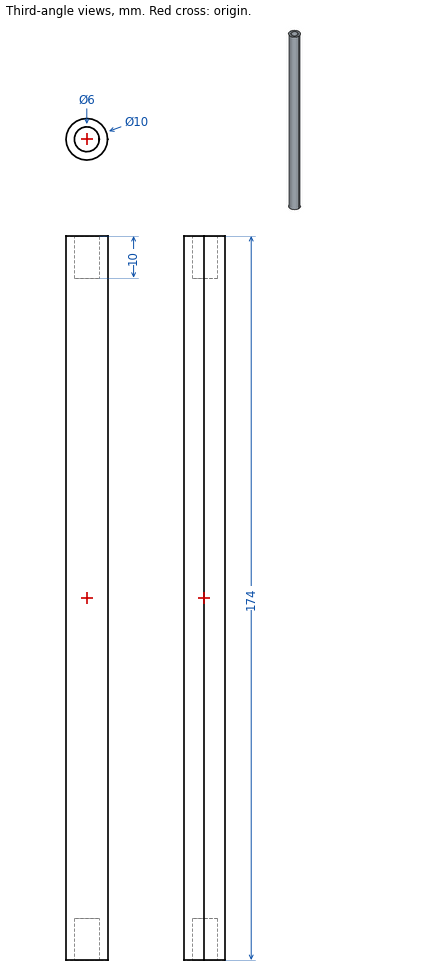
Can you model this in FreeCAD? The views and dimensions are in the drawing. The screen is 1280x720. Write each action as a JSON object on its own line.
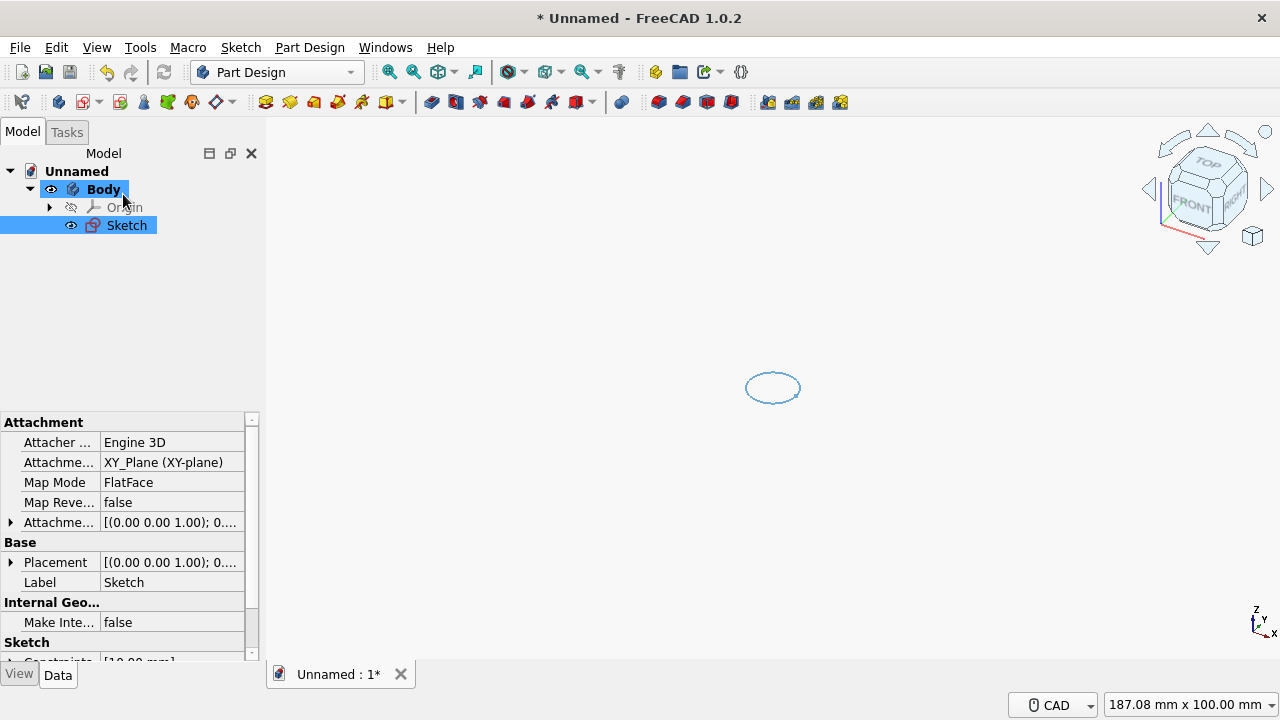
{"action": "left_click", "coordinate": [266, 102]}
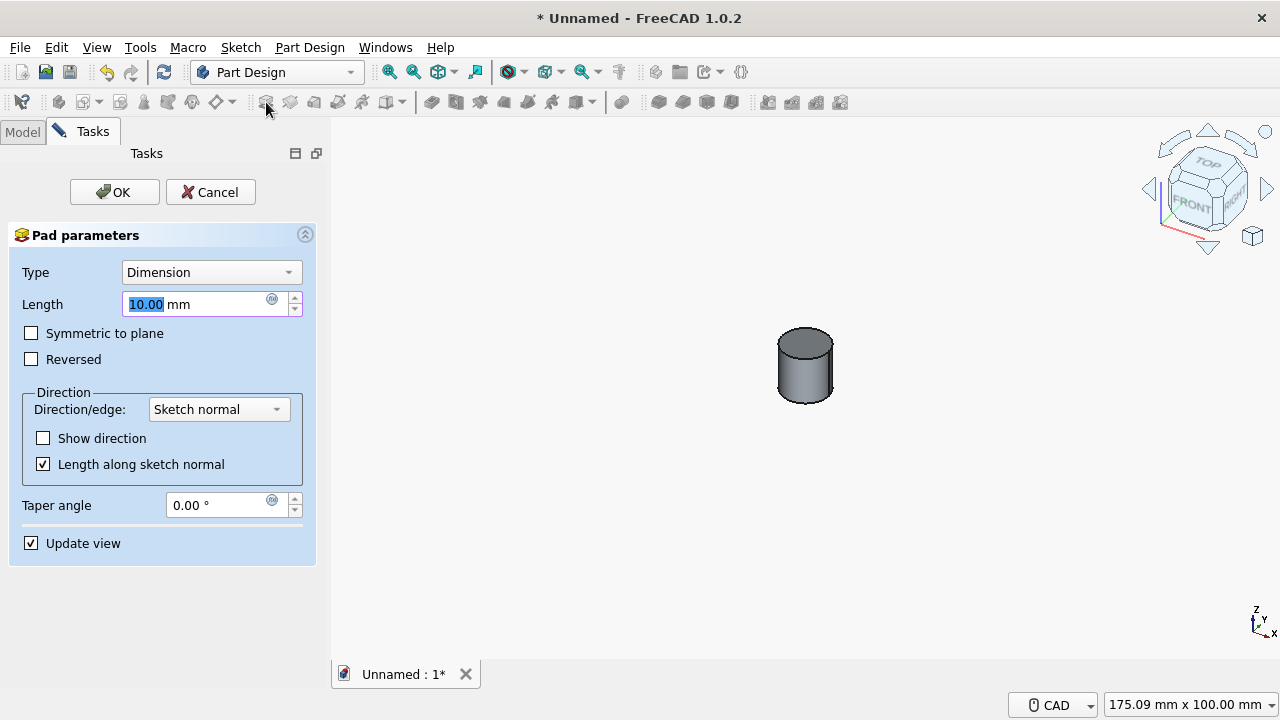
{"action": "type", "text": "174"}
{"action": "key", "text": "Tab"}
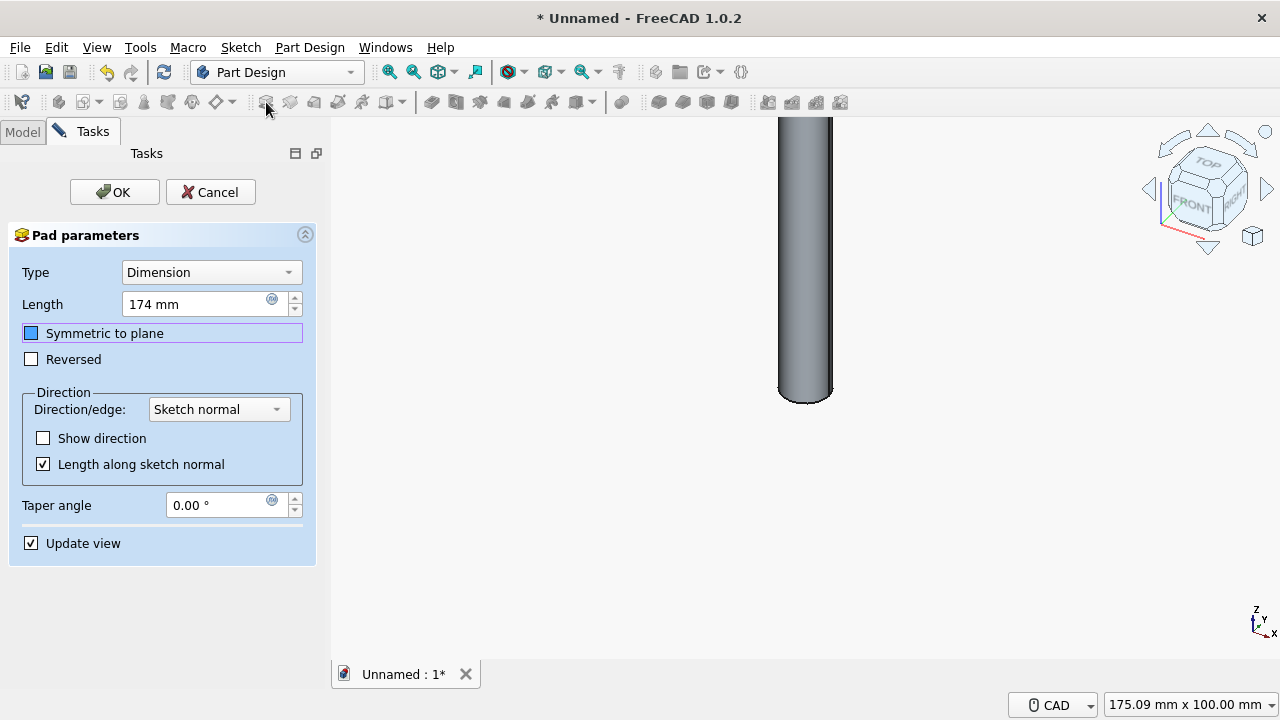
{"action": "left_click", "coordinate": [30, 333]}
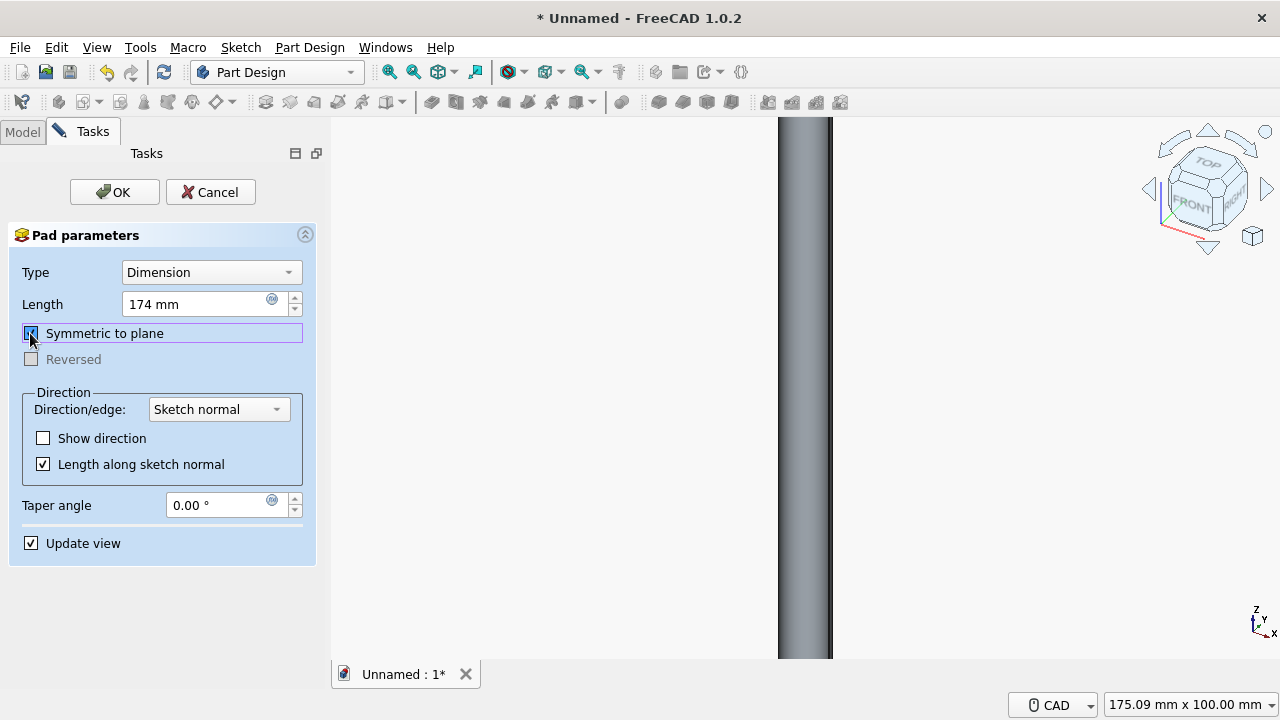
{"action": "left_click", "coordinate": [115, 192]}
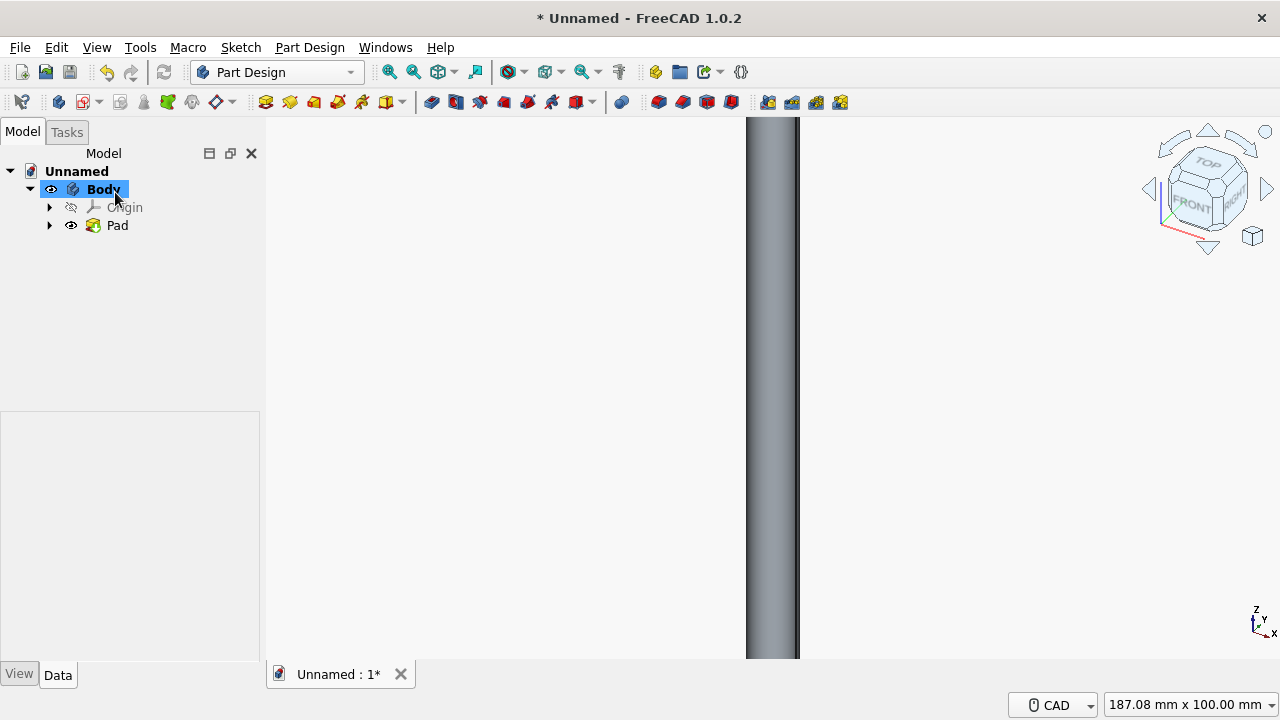
{"action": "left_click", "coordinate": [390, 72]}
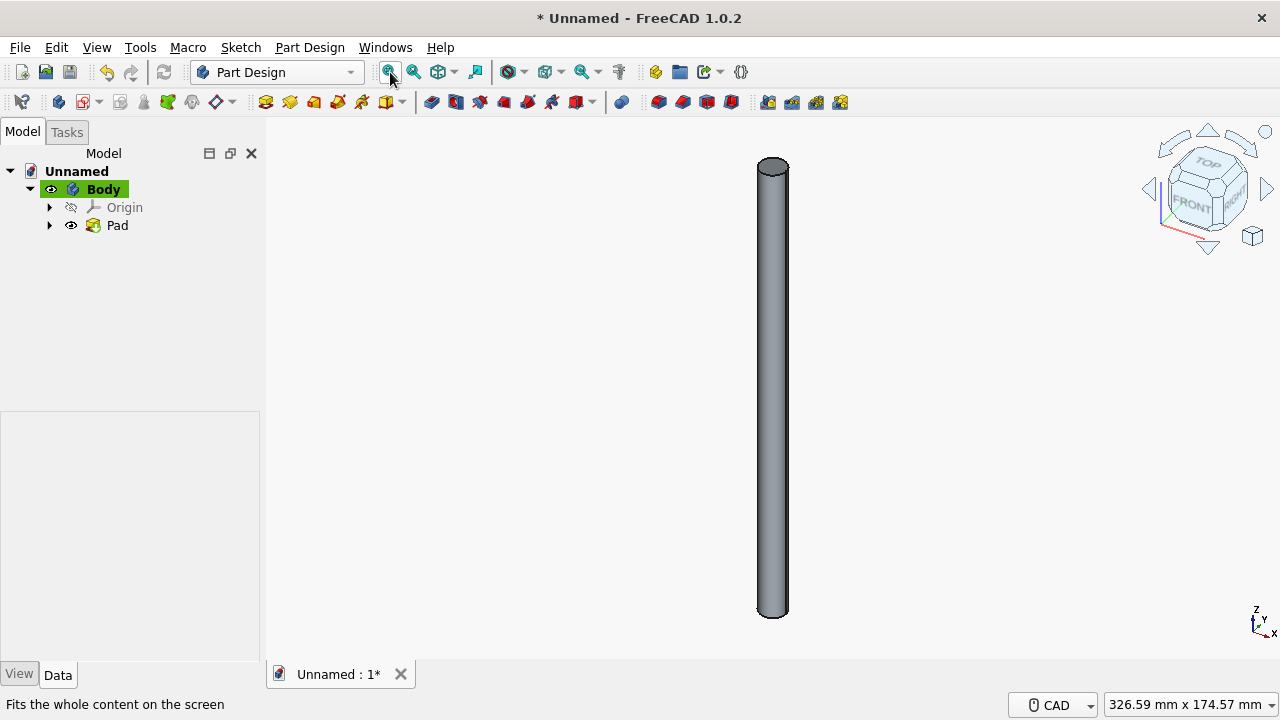
{"action": "left_click", "coordinate": [773, 166]}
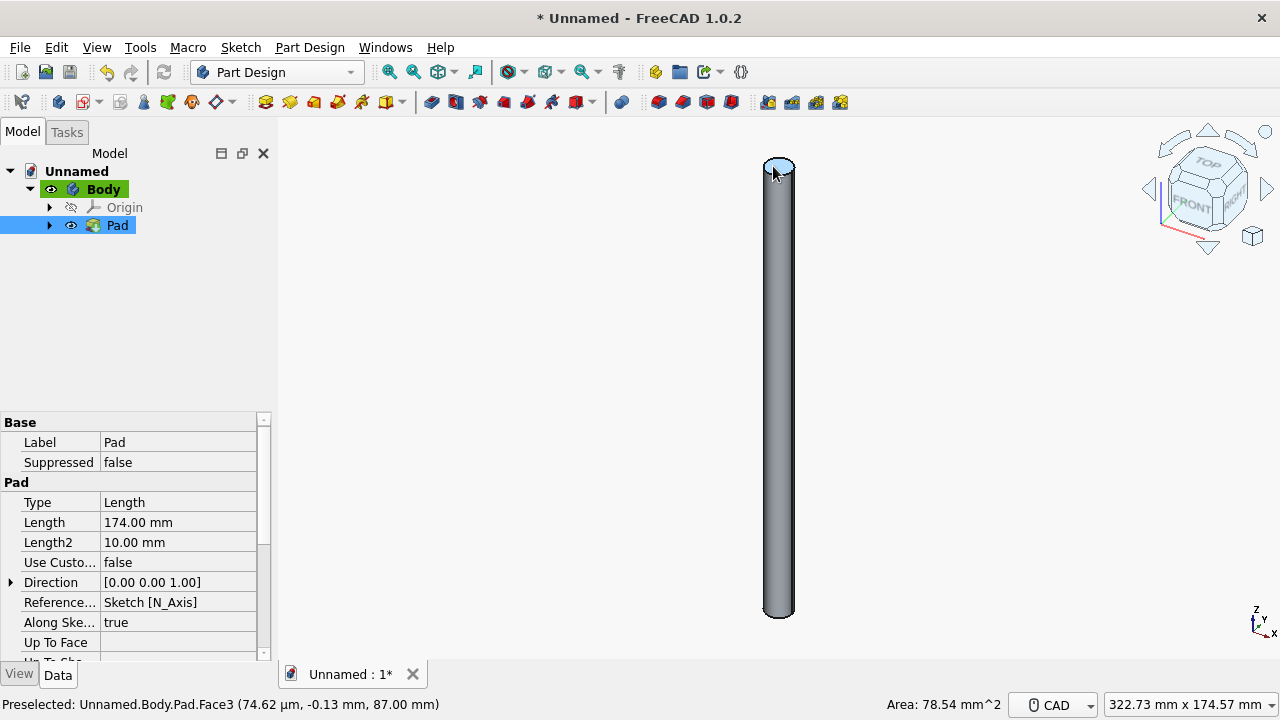
{"action": "left_click", "coordinate": [84, 102]}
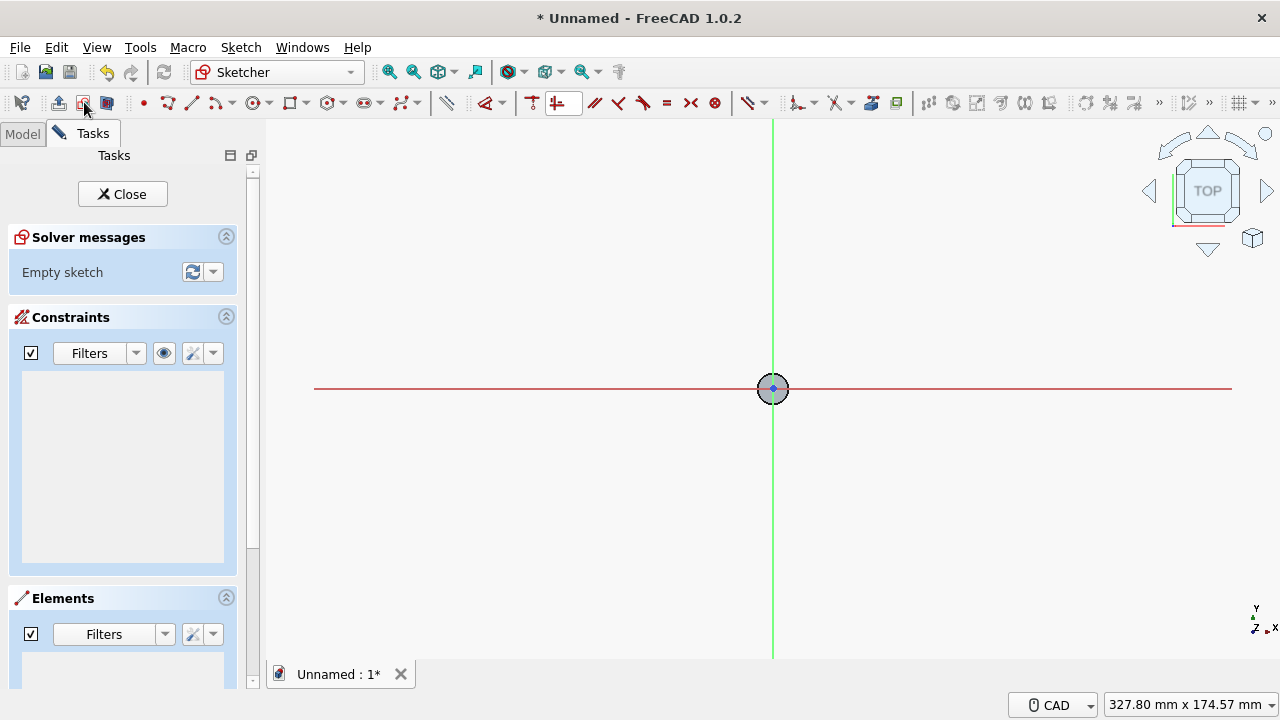
{"action": "scroll", "coordinate": [777, 389], "scroll_direction": "up", "scroll_amount": 15}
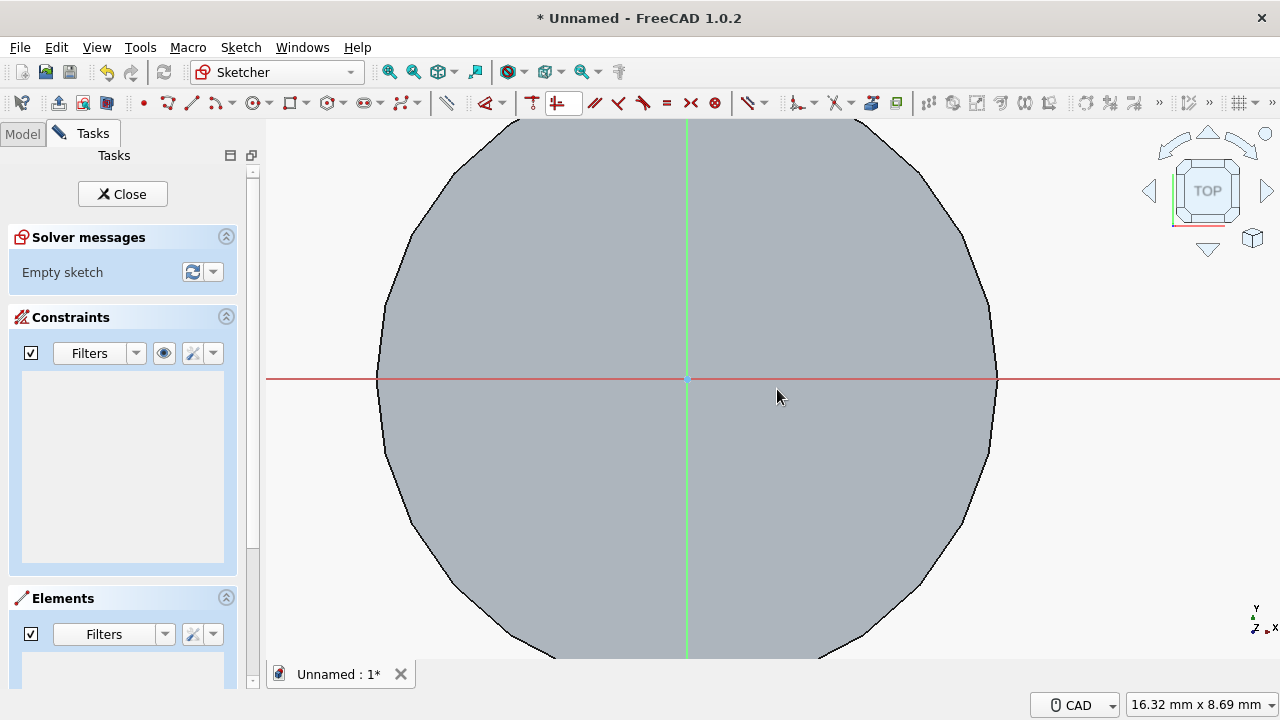
{"action": "left_click", "coordinate": [254, 104]}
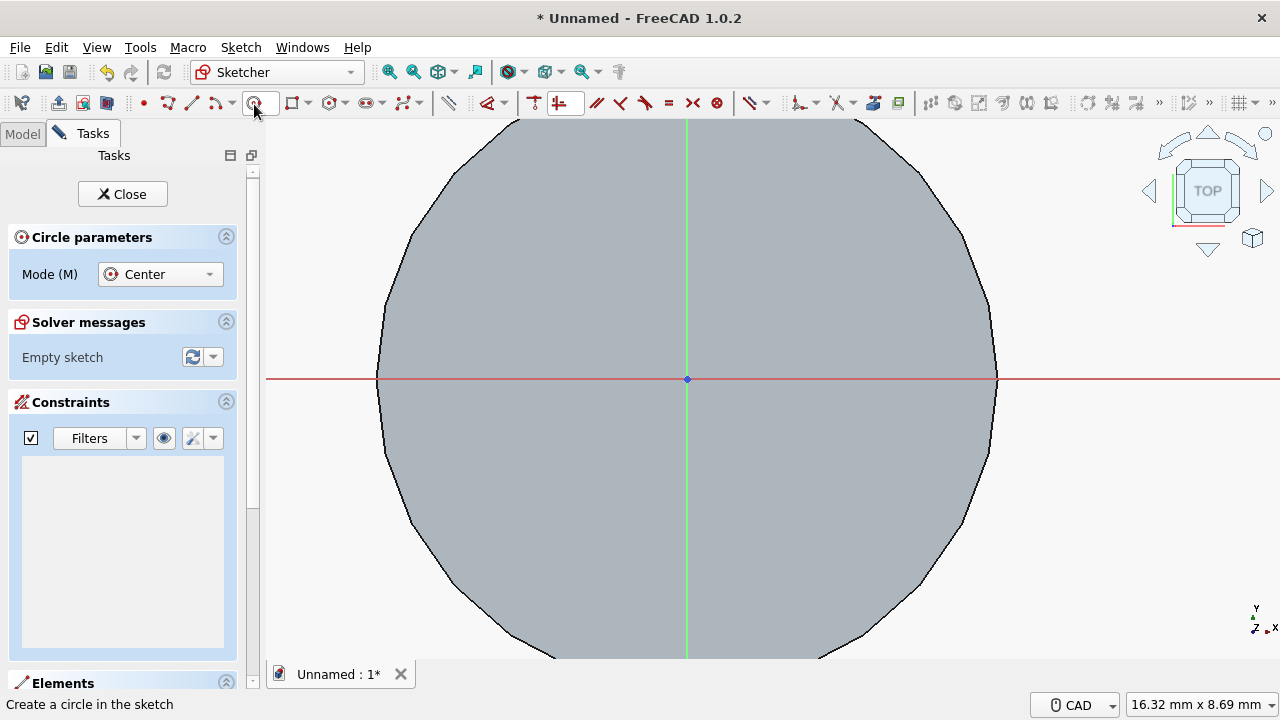
{"action": "left_click", "coordinate": [687, 379]}
{"action": "left_click", "coordinate": [819, 248]}
{"action": "key", "text": "Escape"}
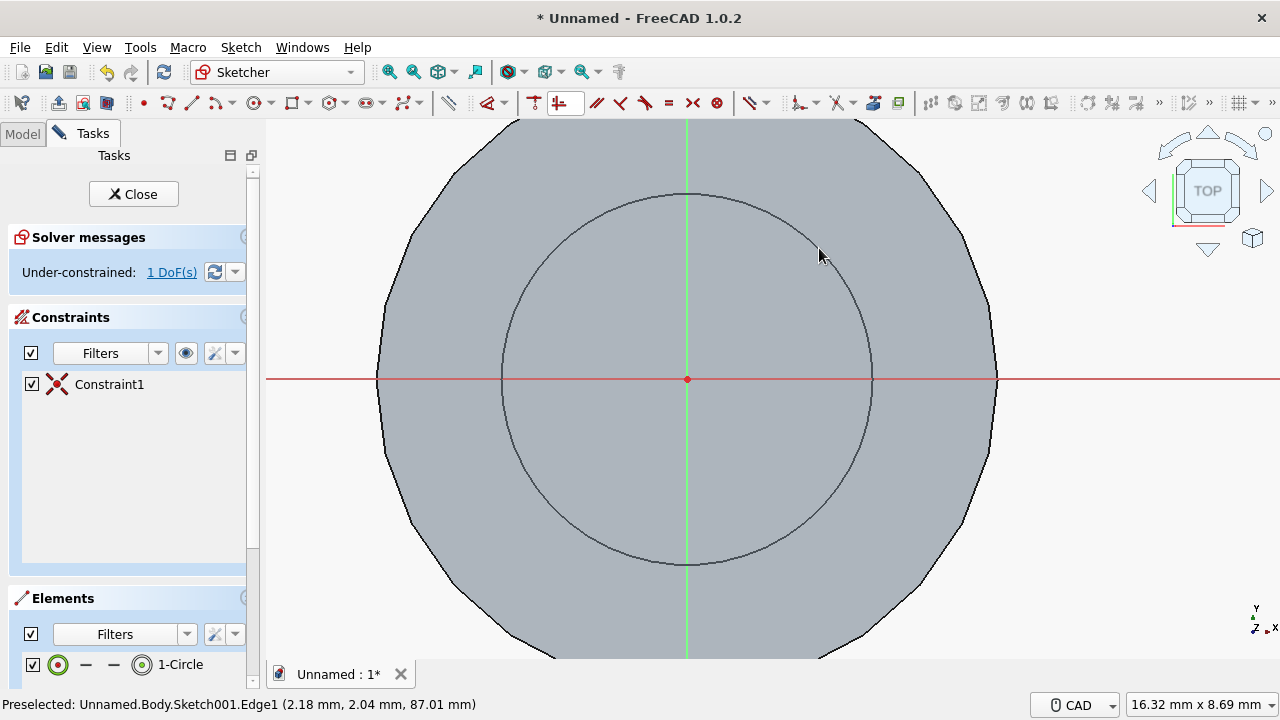
{"action": "left_click", "coordinate": [488, 104]}